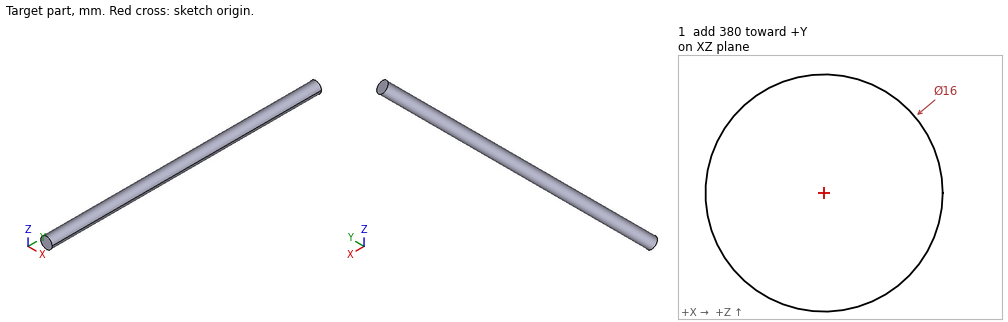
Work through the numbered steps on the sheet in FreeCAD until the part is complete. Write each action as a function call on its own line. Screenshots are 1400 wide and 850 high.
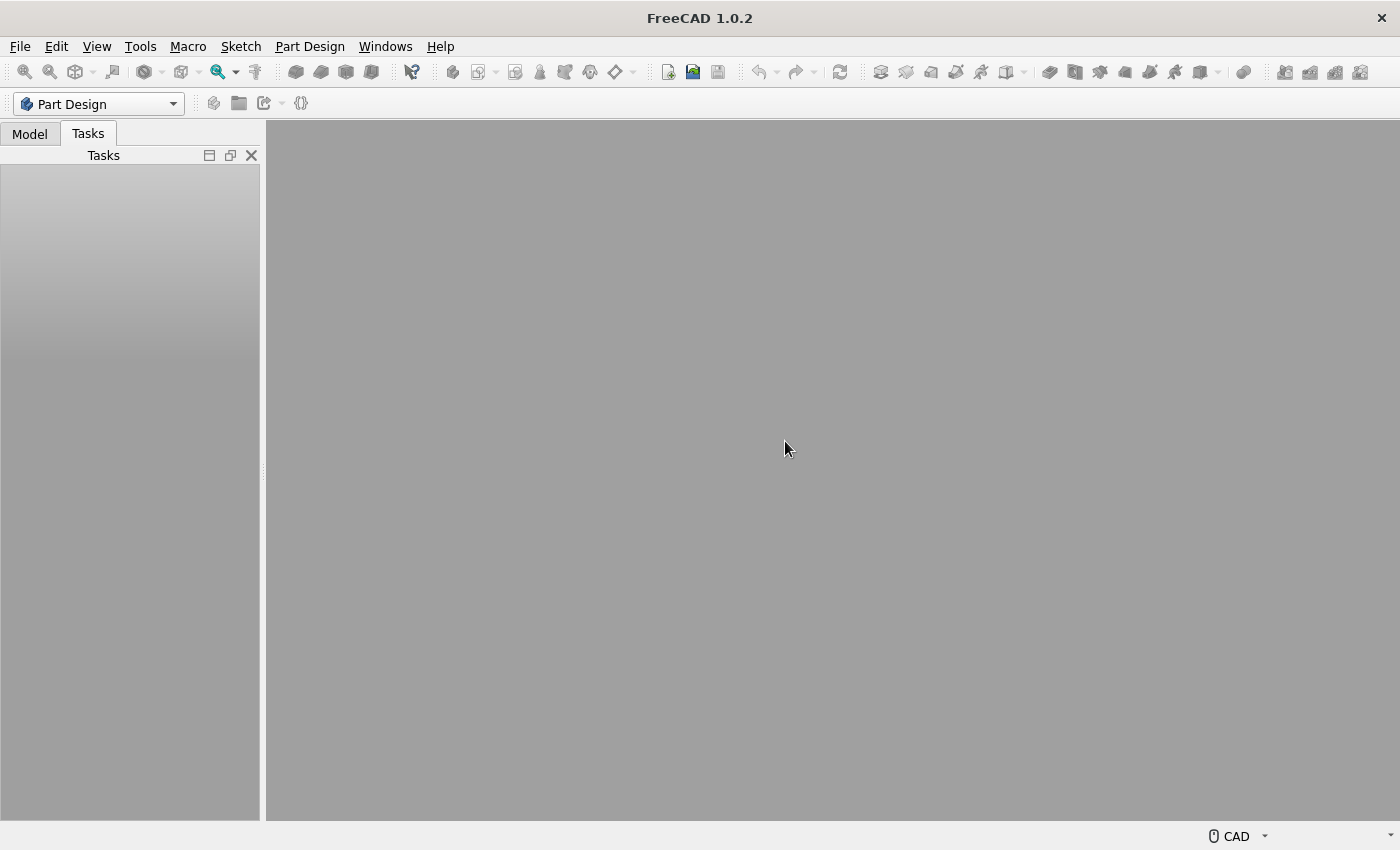
key(ctrl+n)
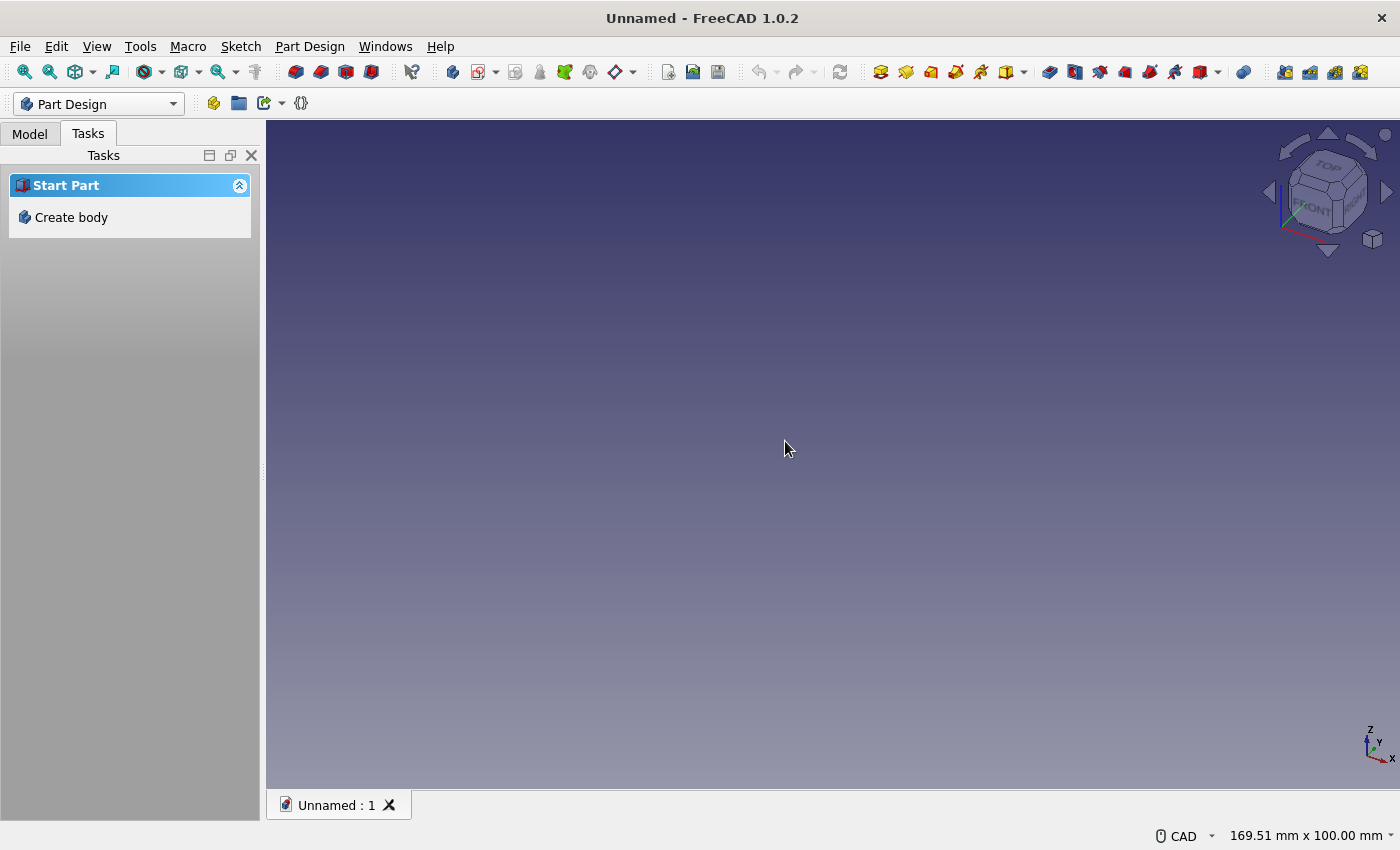
click(478, 72)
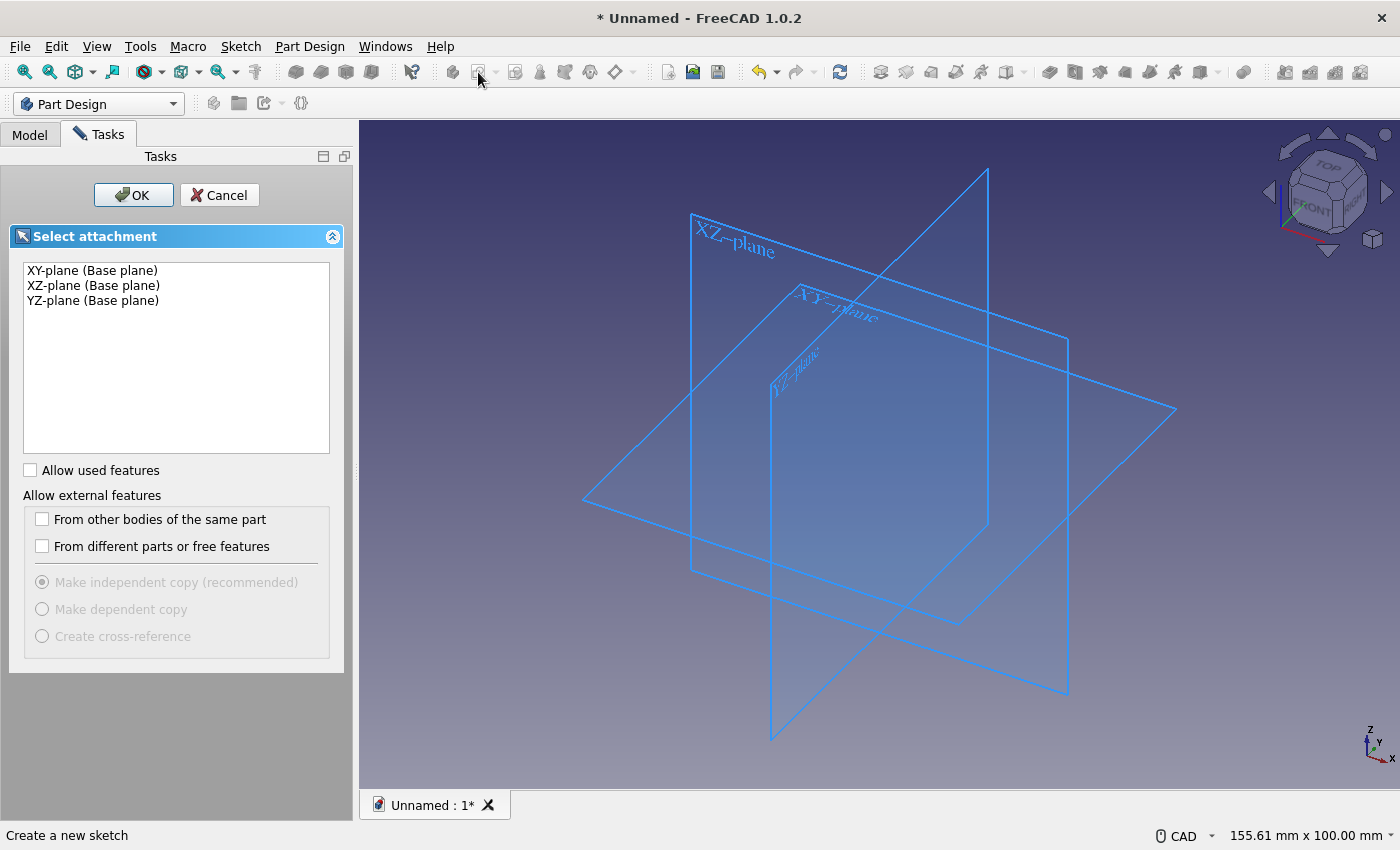
click(84, 286)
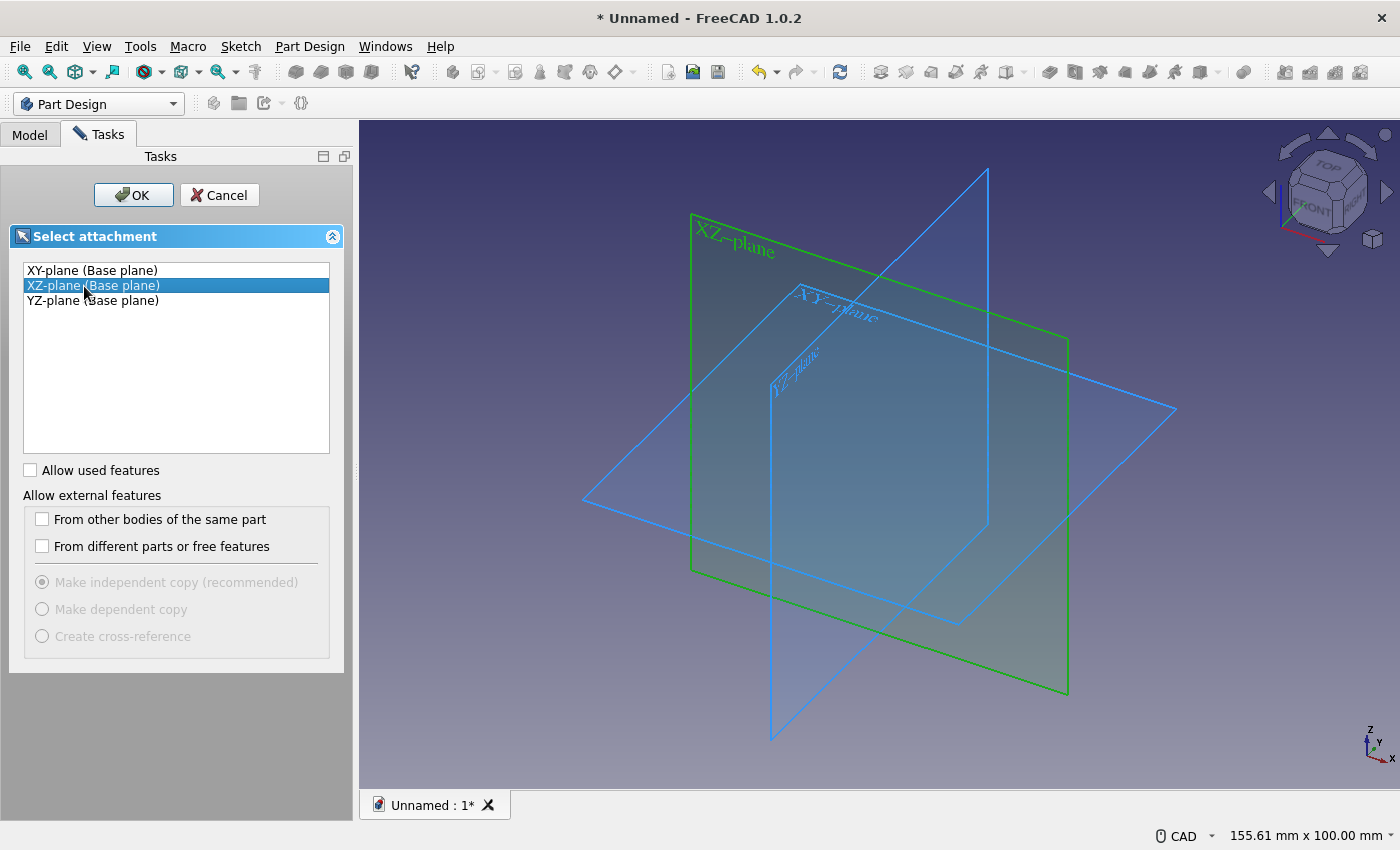
click(134, 195)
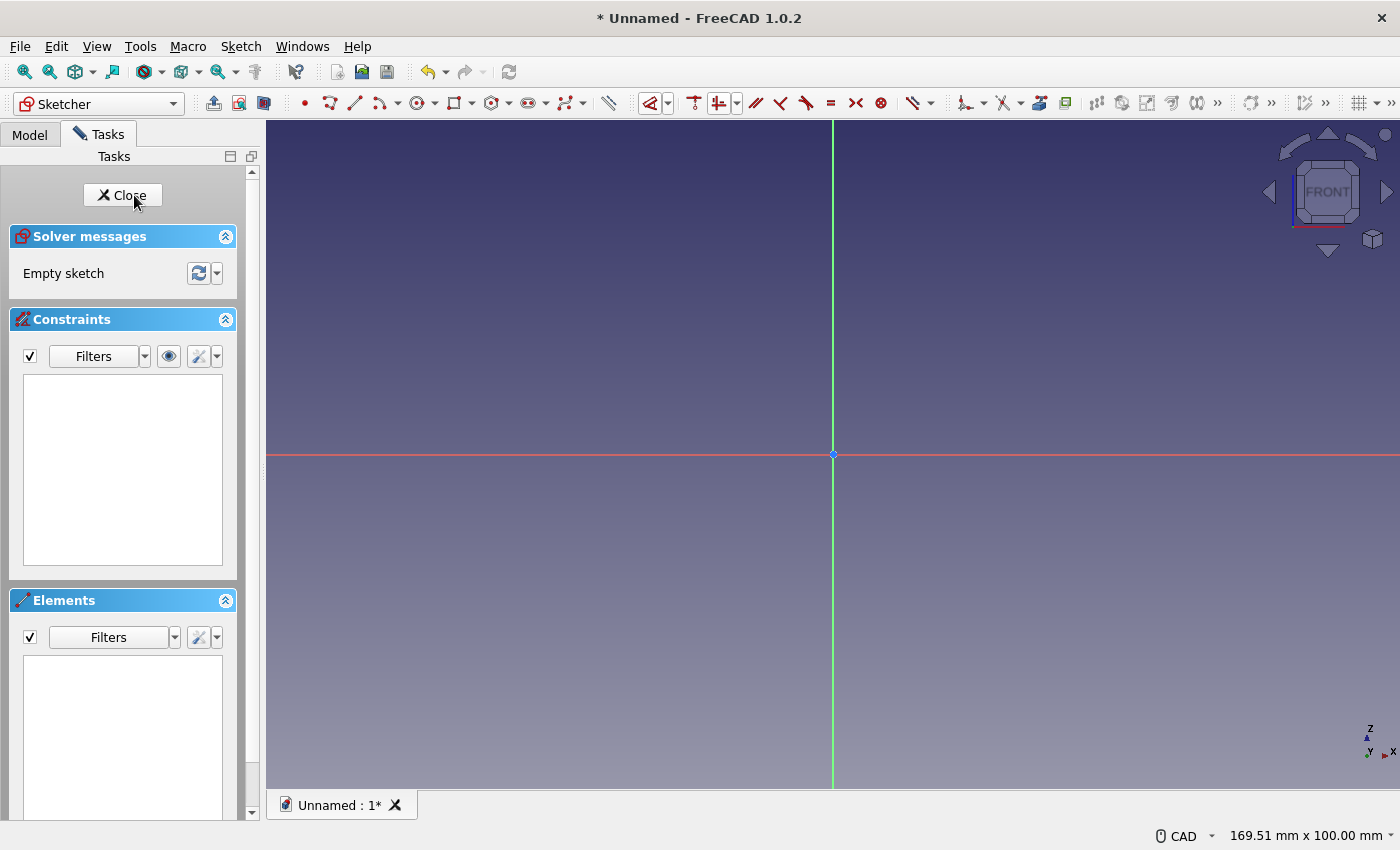
scroll(855, 454, up, 7)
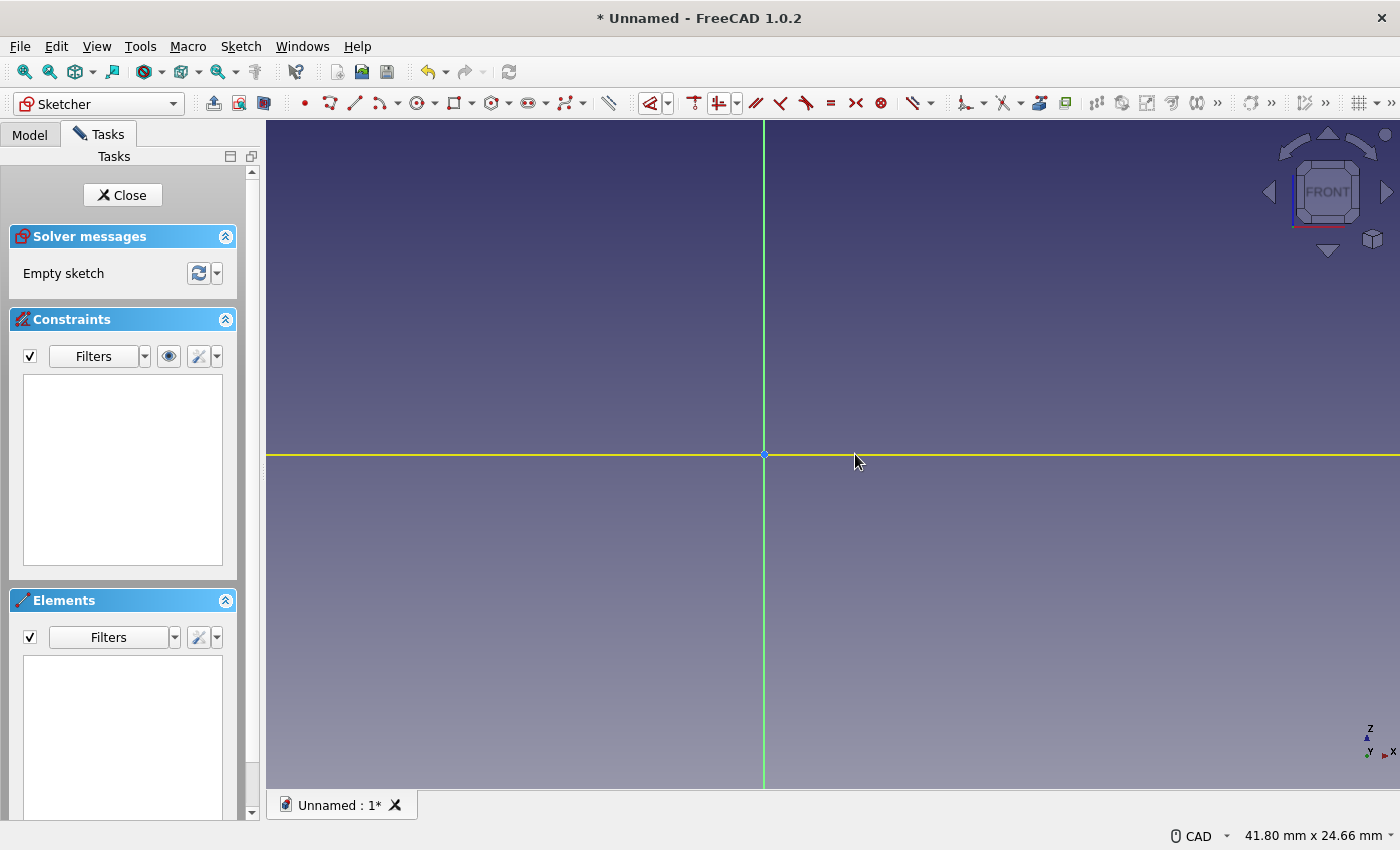
key(g)
key(c)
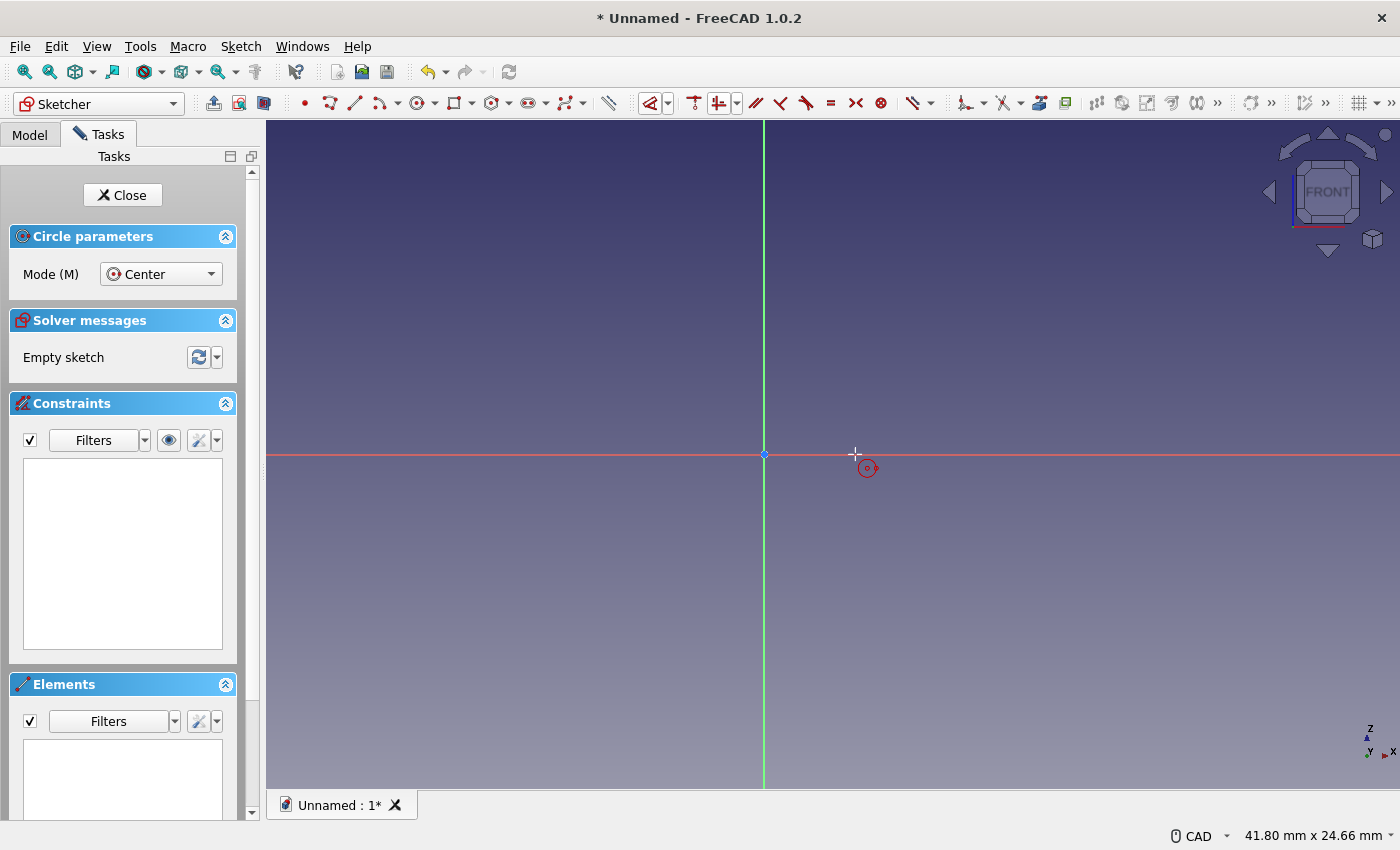
click(764, 454)
move(918, 301)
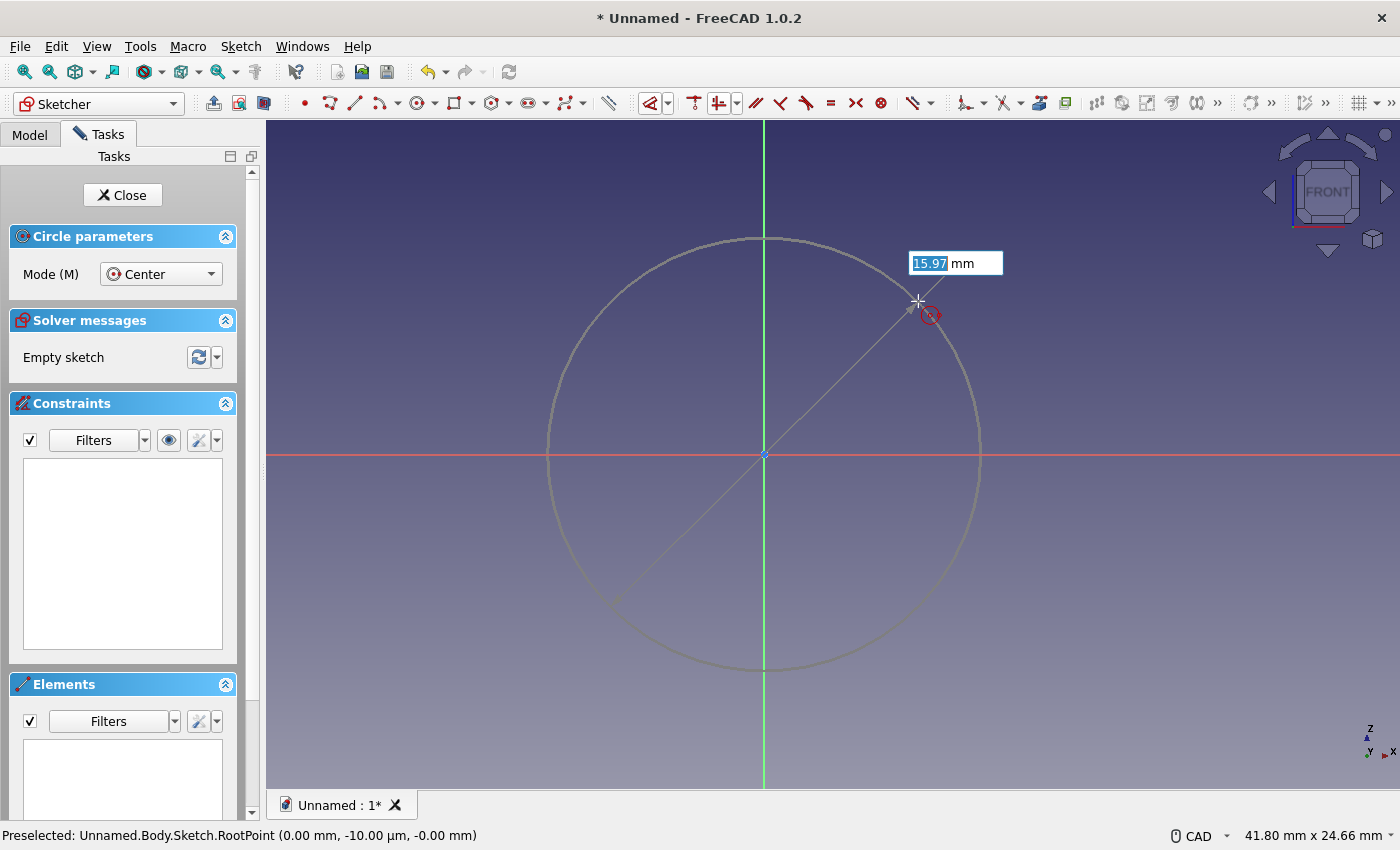
text(16)
key(Return)
key(Escape)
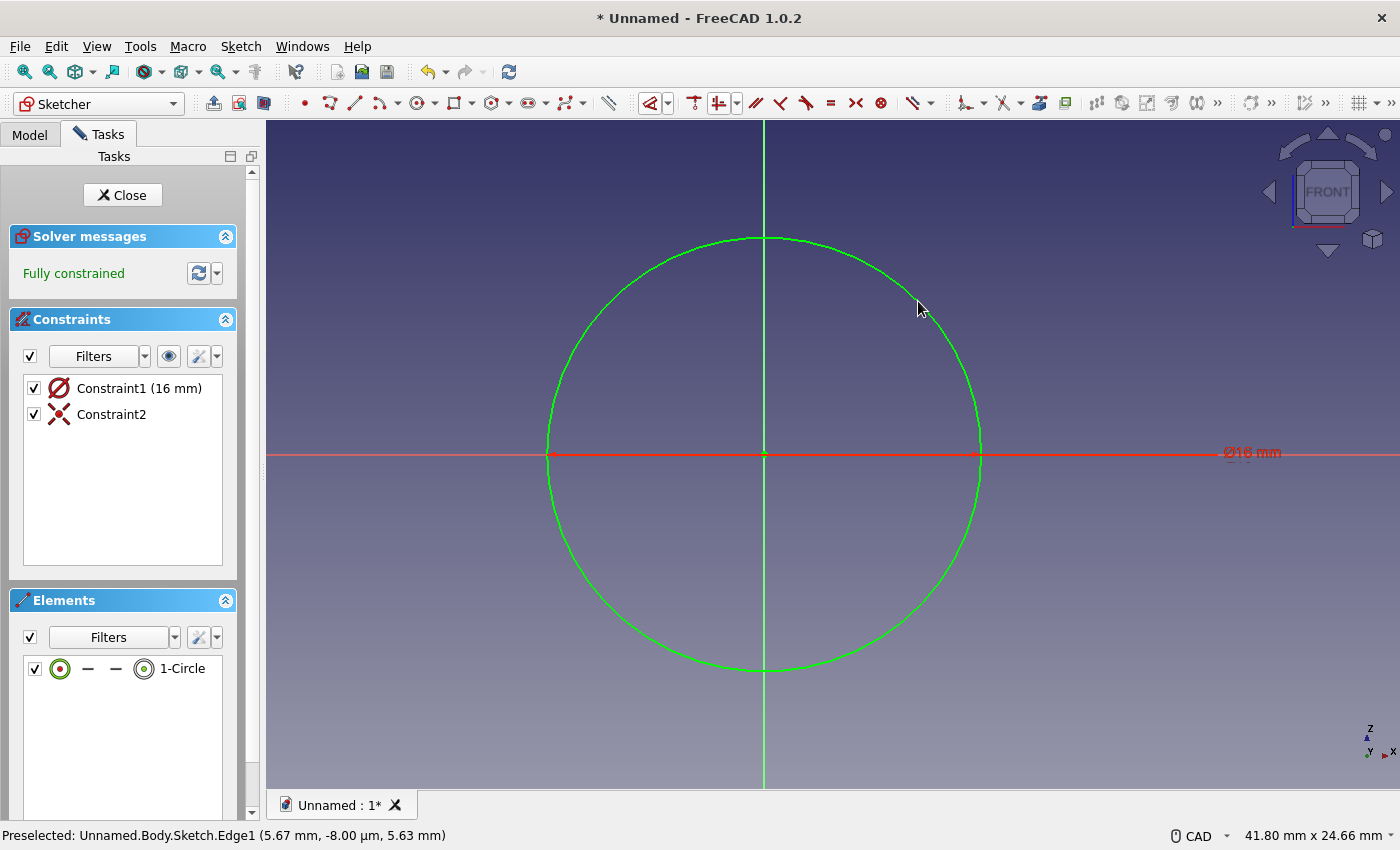
click(123, 195)